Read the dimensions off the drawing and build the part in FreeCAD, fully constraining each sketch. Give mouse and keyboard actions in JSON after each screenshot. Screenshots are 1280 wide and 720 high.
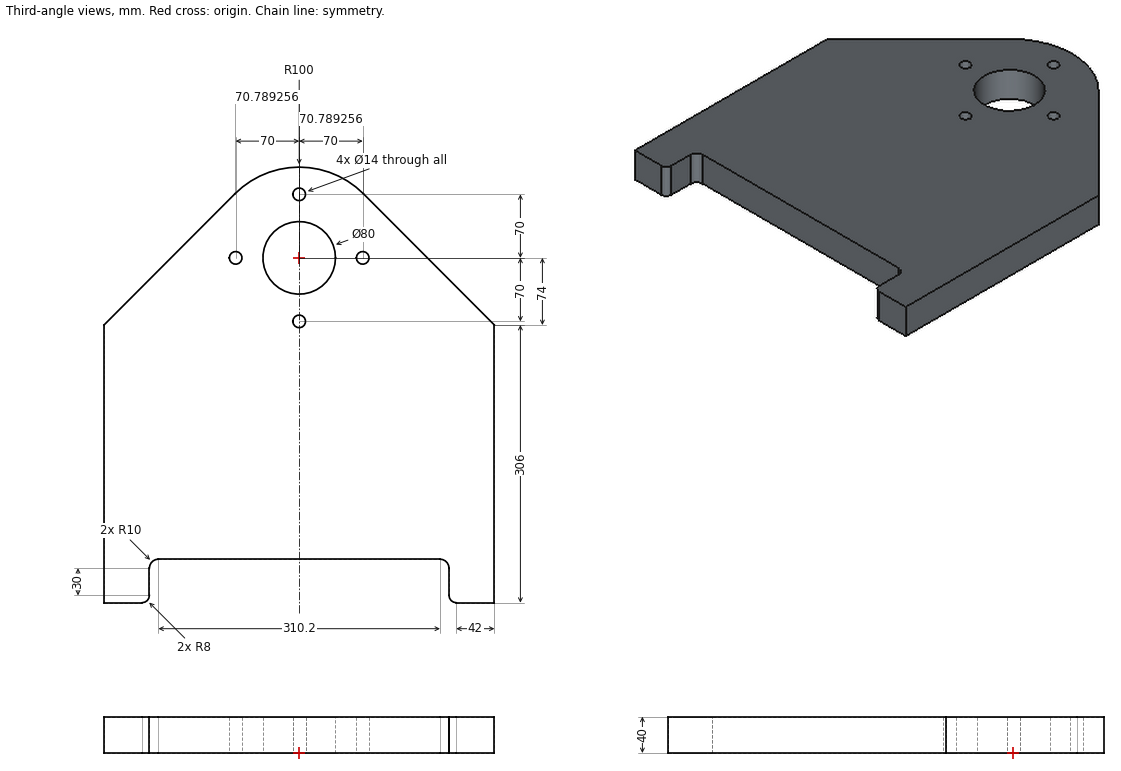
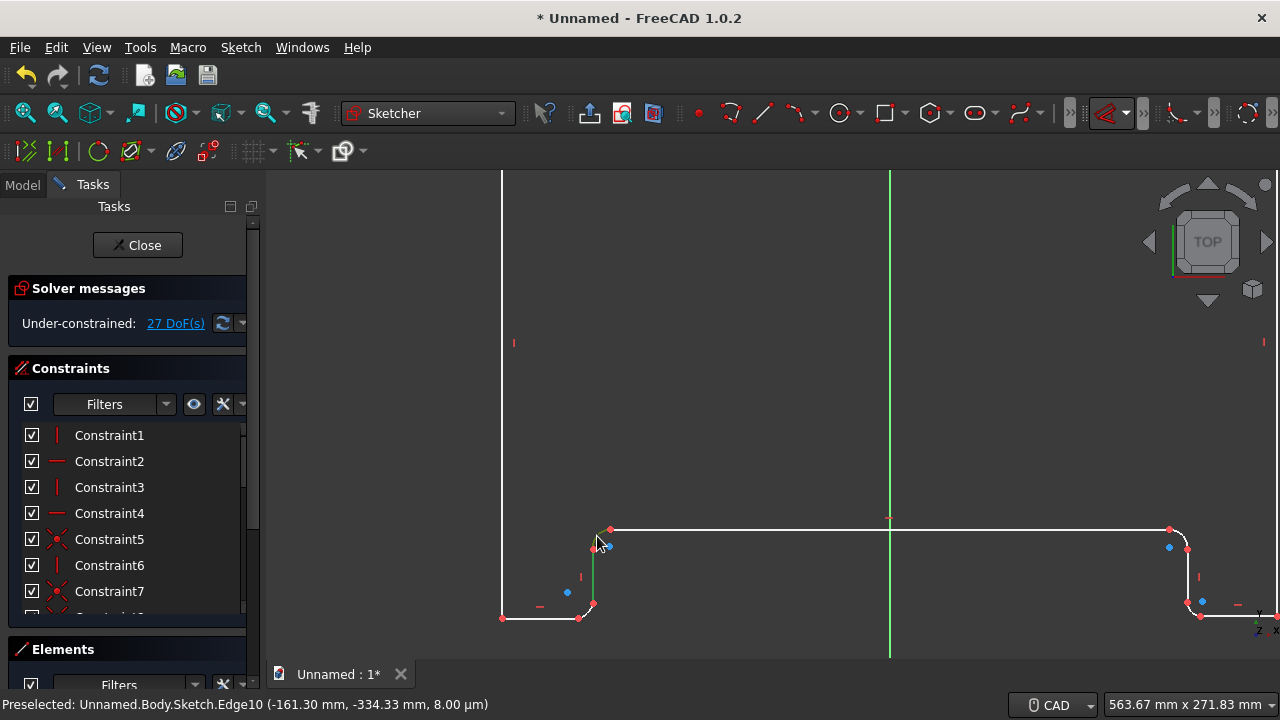
{"action": "key", "text": "t"}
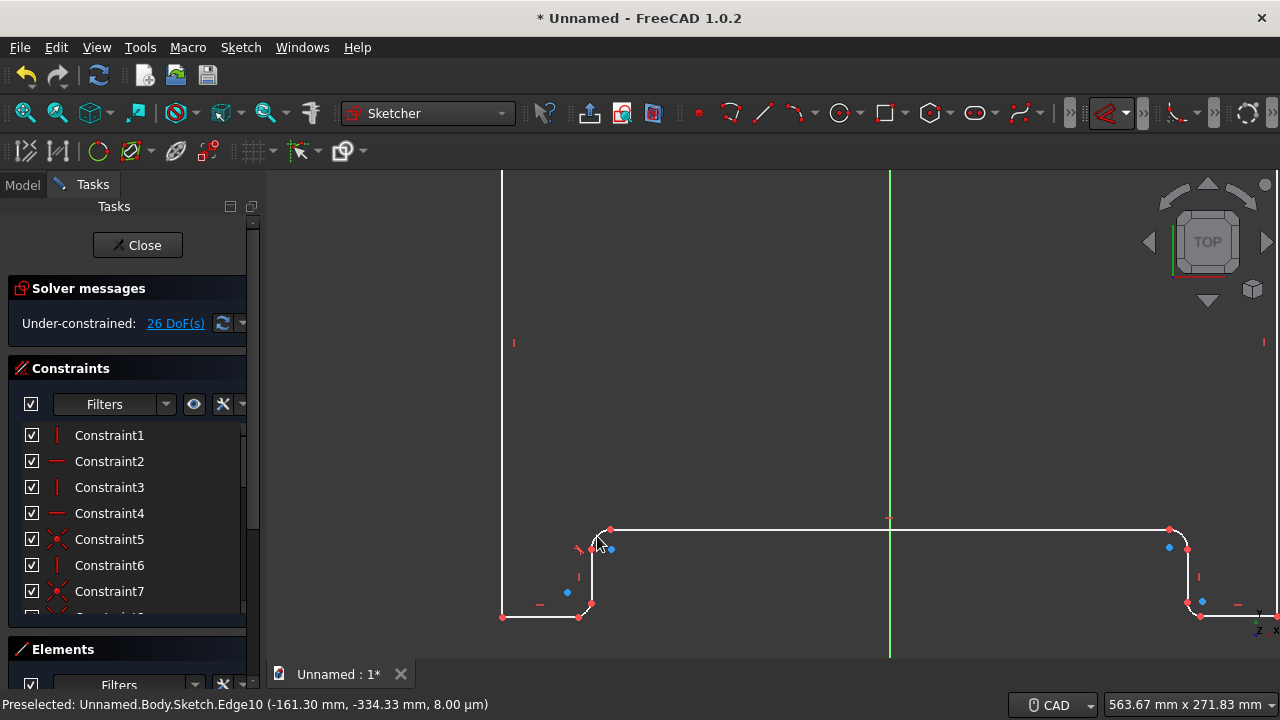
{"action": "left_click", "coordinate": [592, 587]}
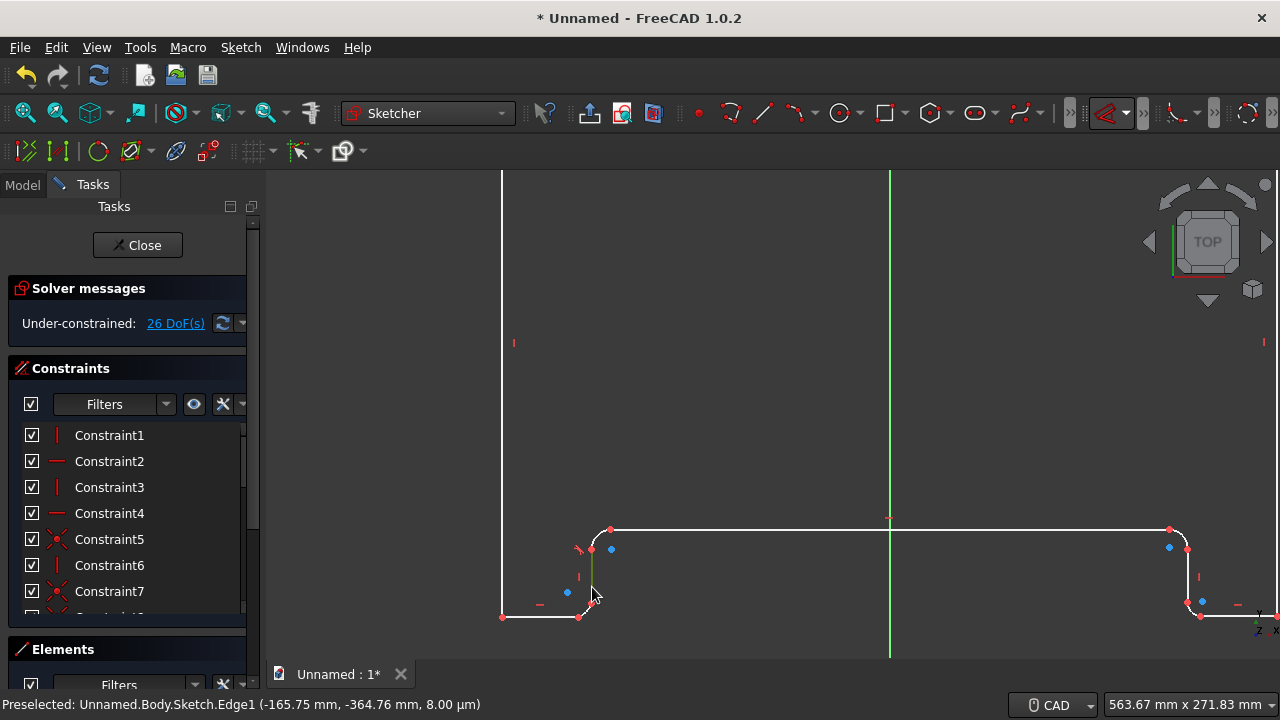
{"action": "scroll", "coordinate": [586, 612], "scroll_direction": "up", "scroll_amount": 2}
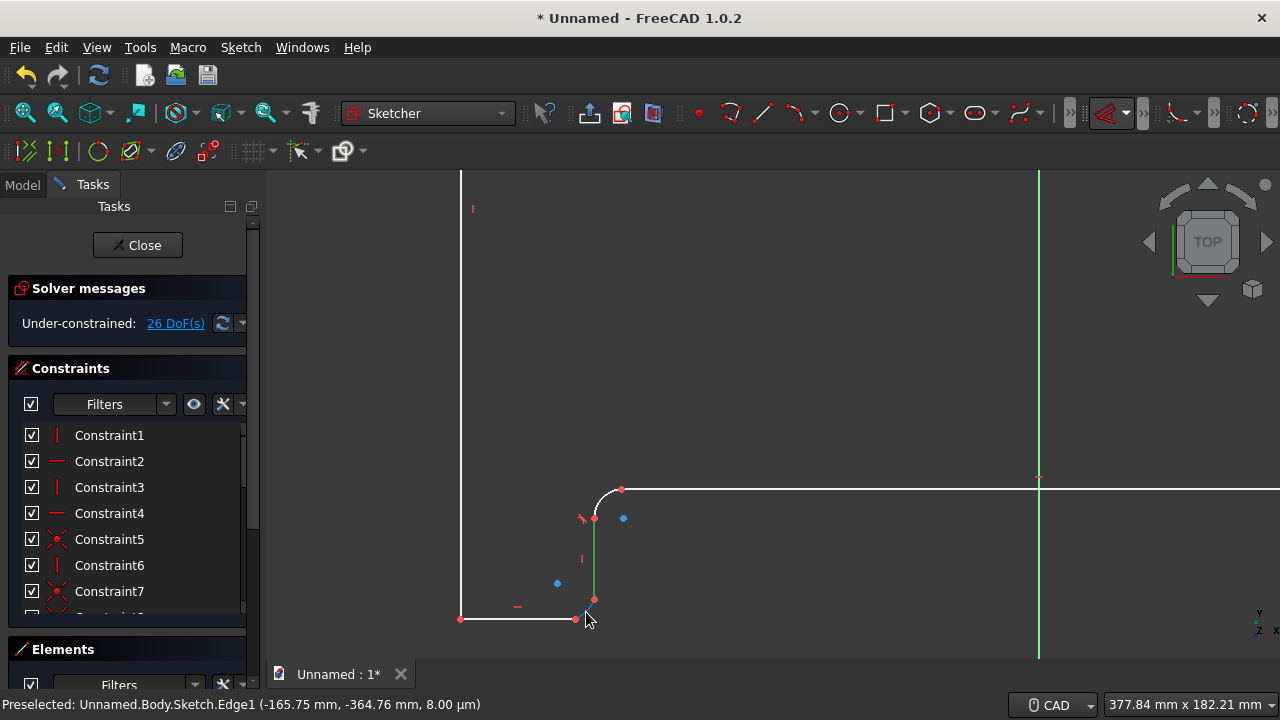
{"action": "left_click", "coordinate": [587, 611]}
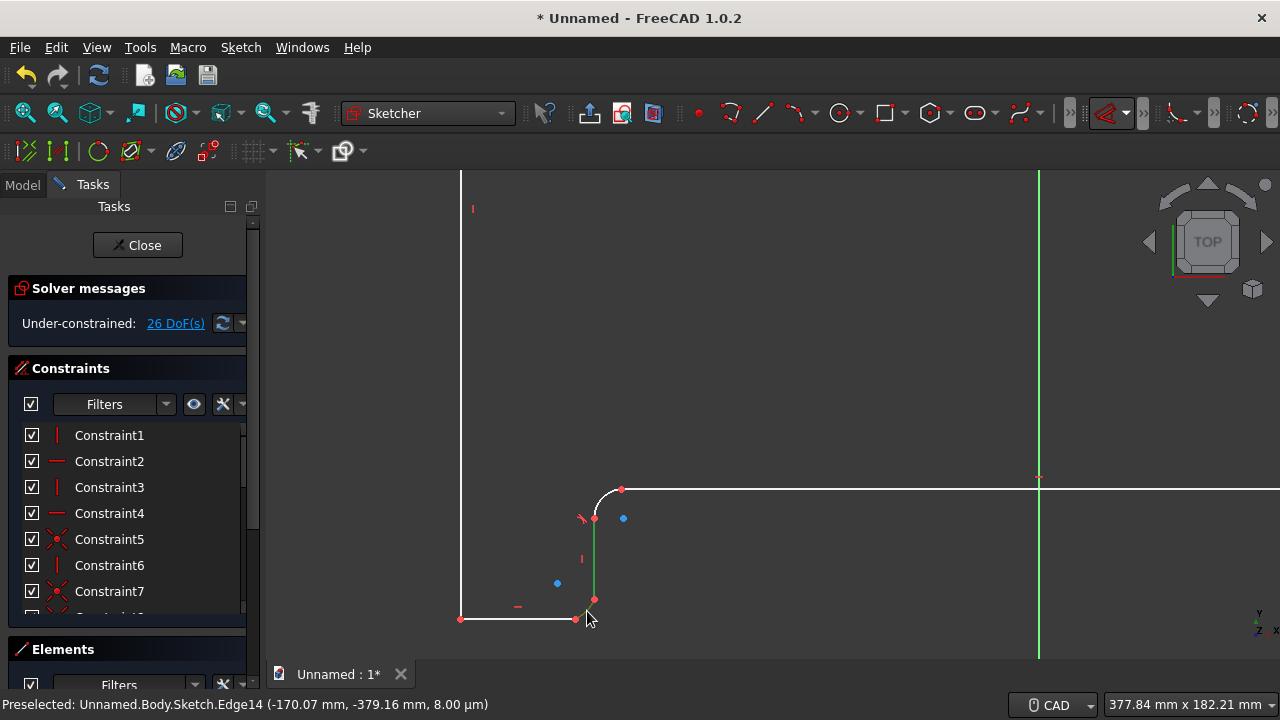
{"action": "key", "text": "t"}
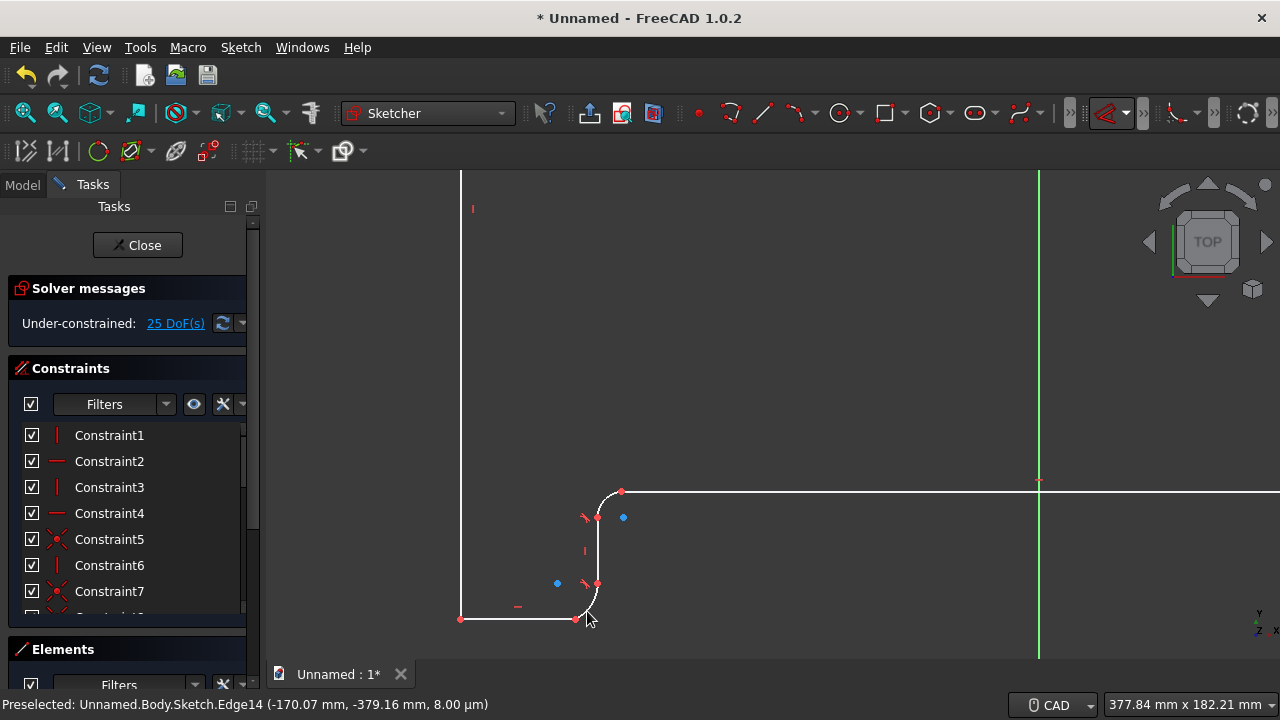
{"action": "scroll", "coordinate": [595, 559], "scroll_direction": "down", "scroll_amount": 7}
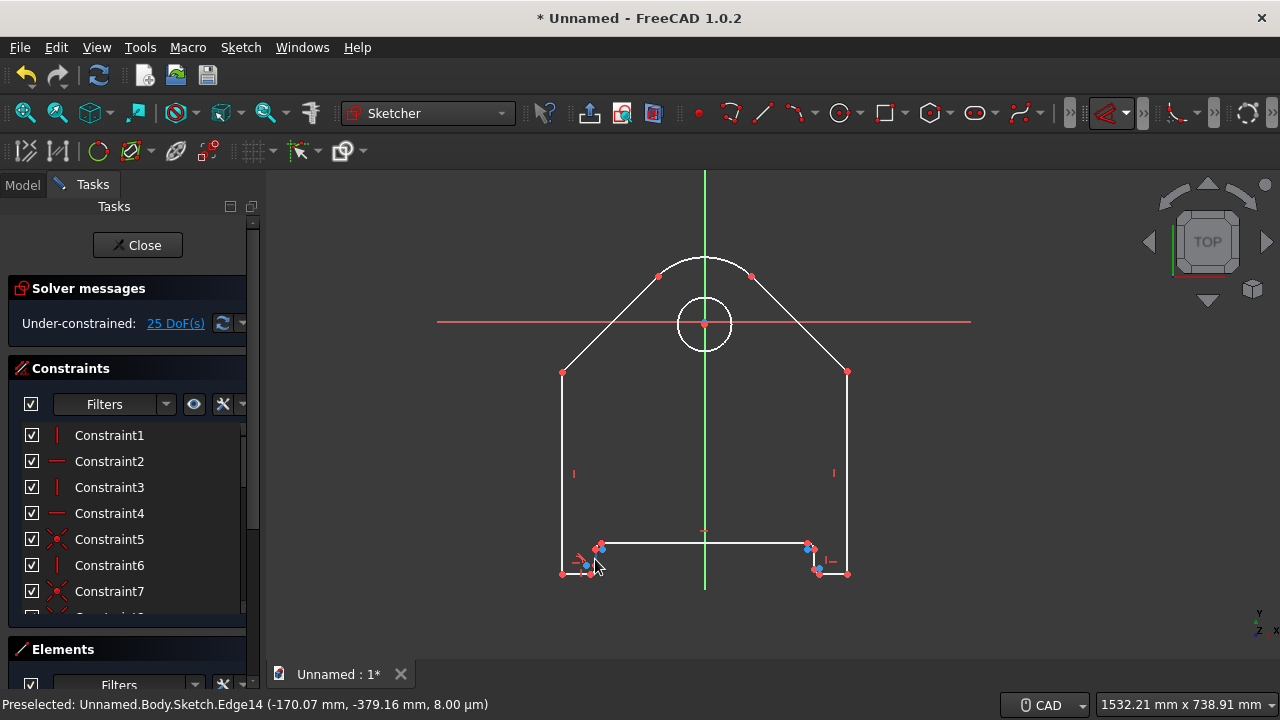
{"action": "left_click", "coordinate": [664, 543]}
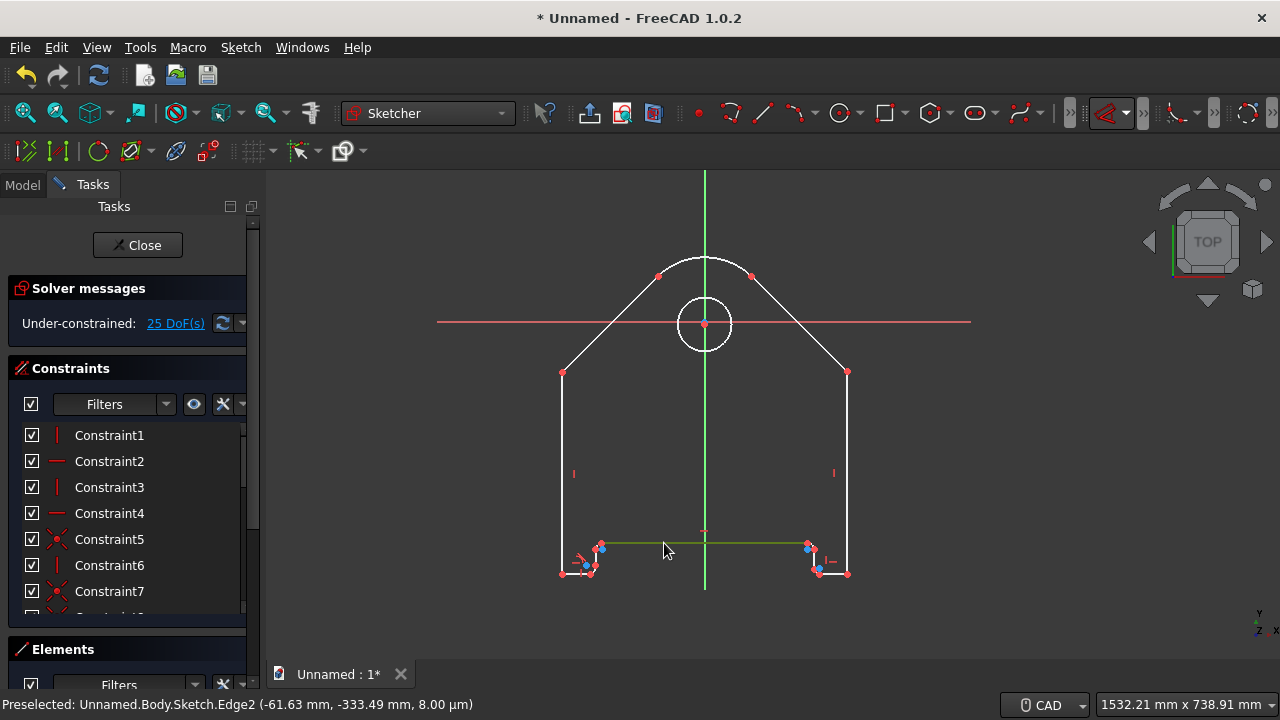
{"action": "scroll", "coordinate": [598, 545], "scroll_direction": "up", "scroll_amount": 6}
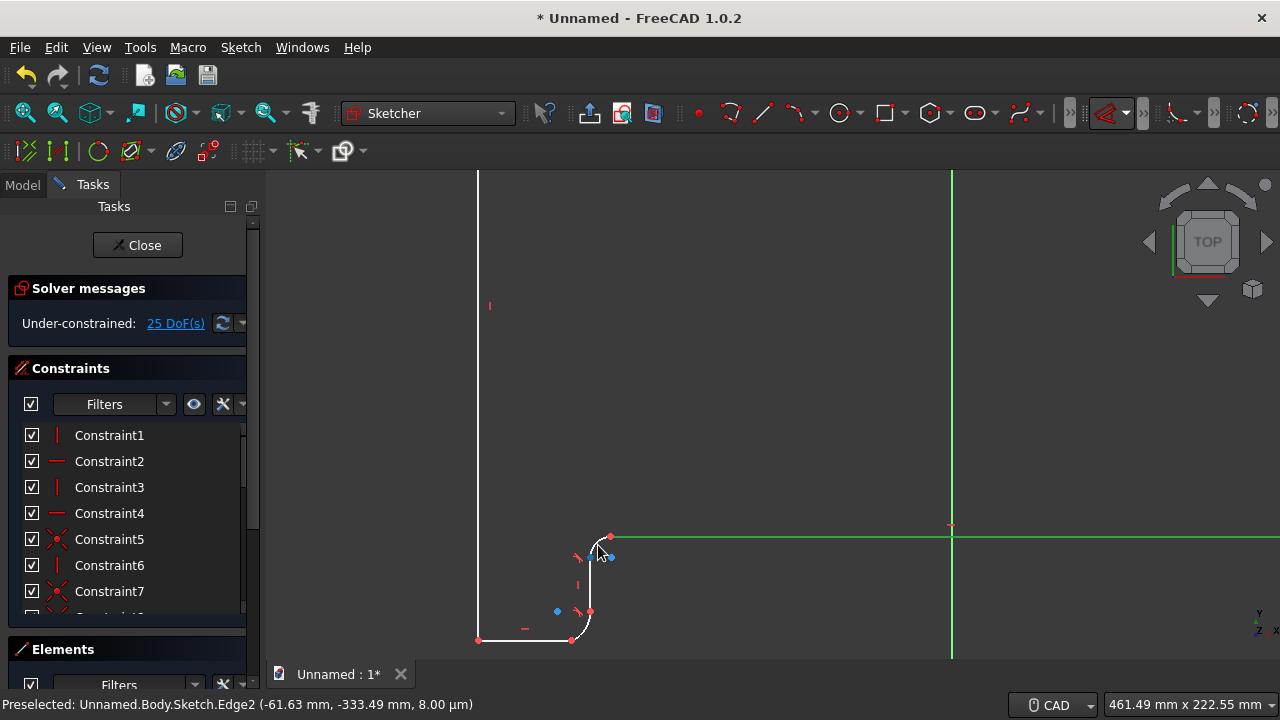
{"action": "left_click", "coordinate": [596, 543]}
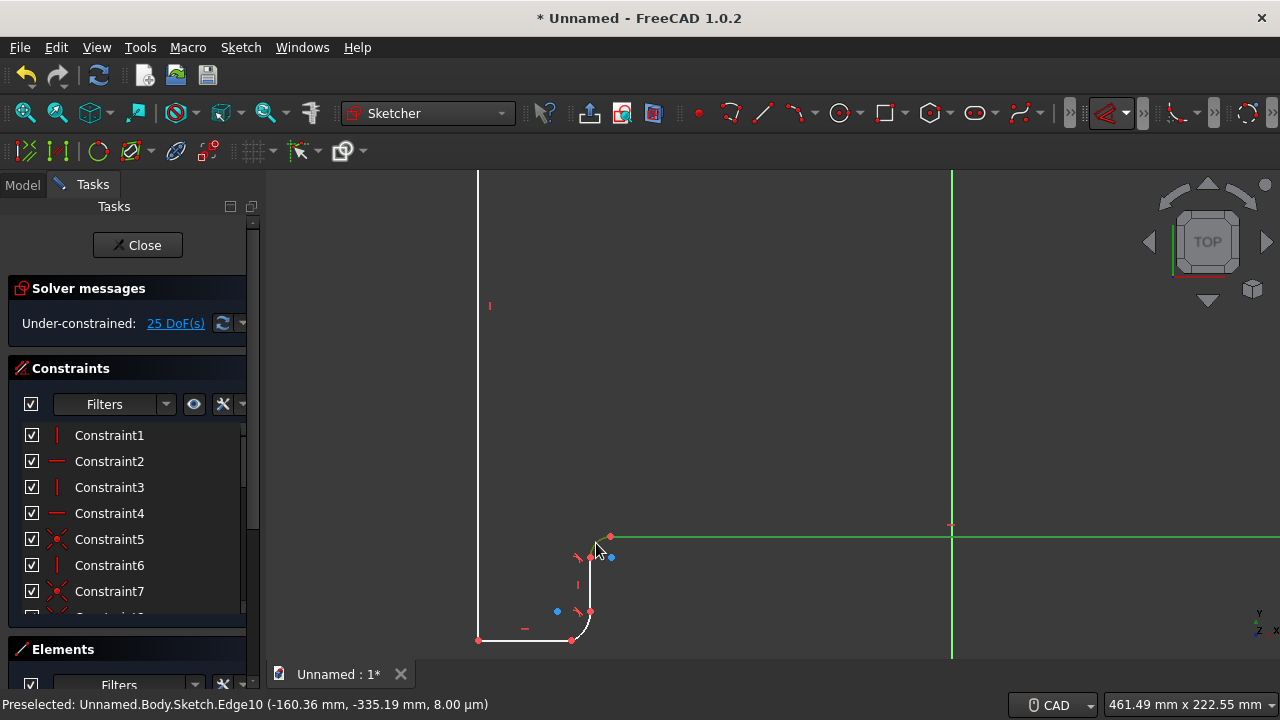
{"action": "key", "text": "t"}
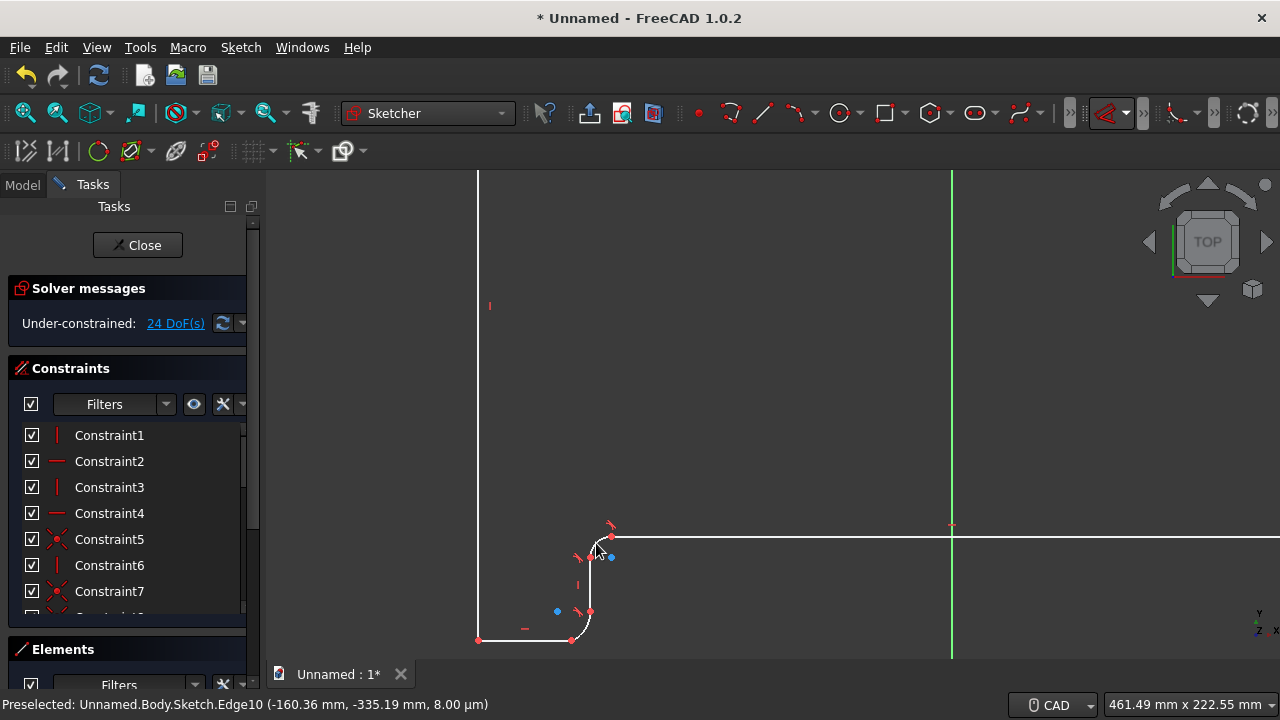
{"action": "left_click", "coordinate": [816, 537]}